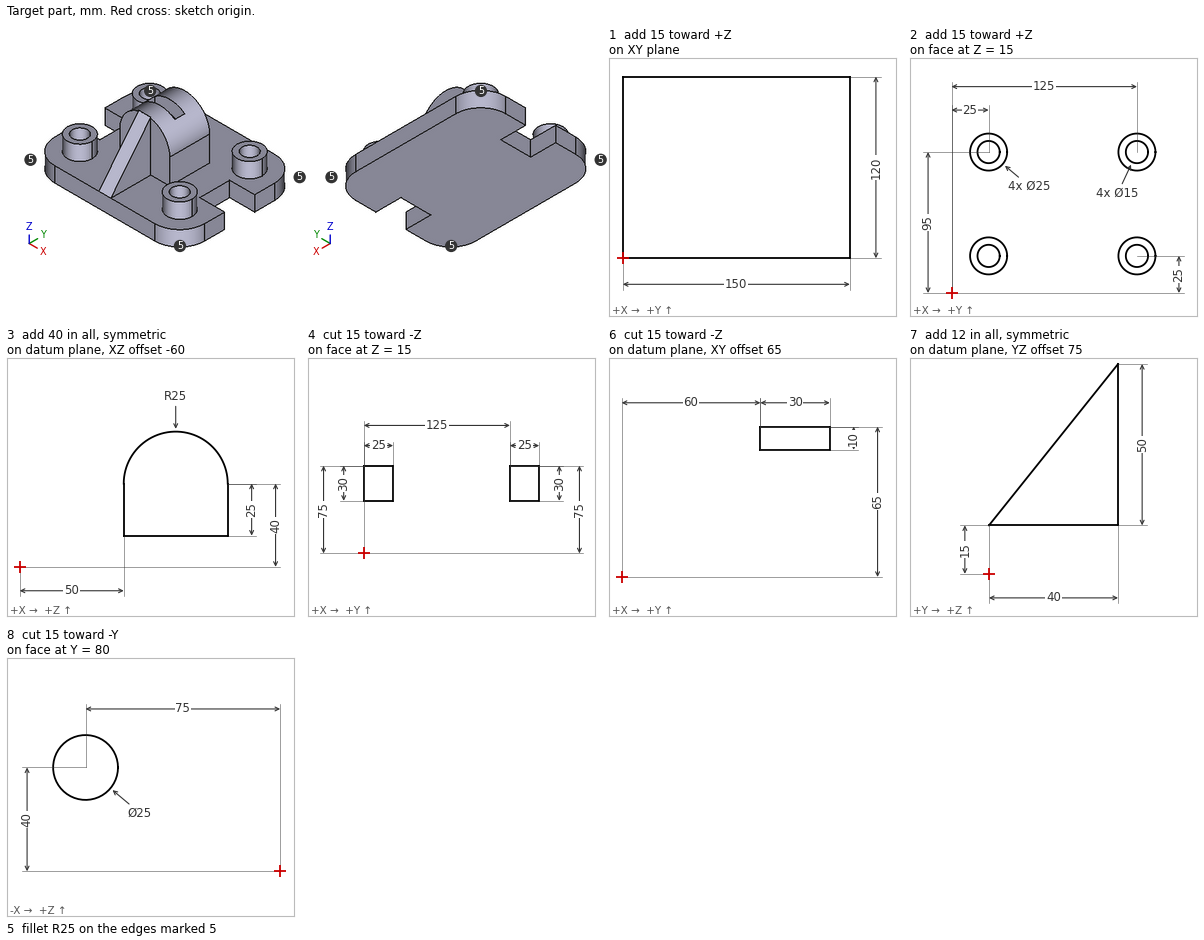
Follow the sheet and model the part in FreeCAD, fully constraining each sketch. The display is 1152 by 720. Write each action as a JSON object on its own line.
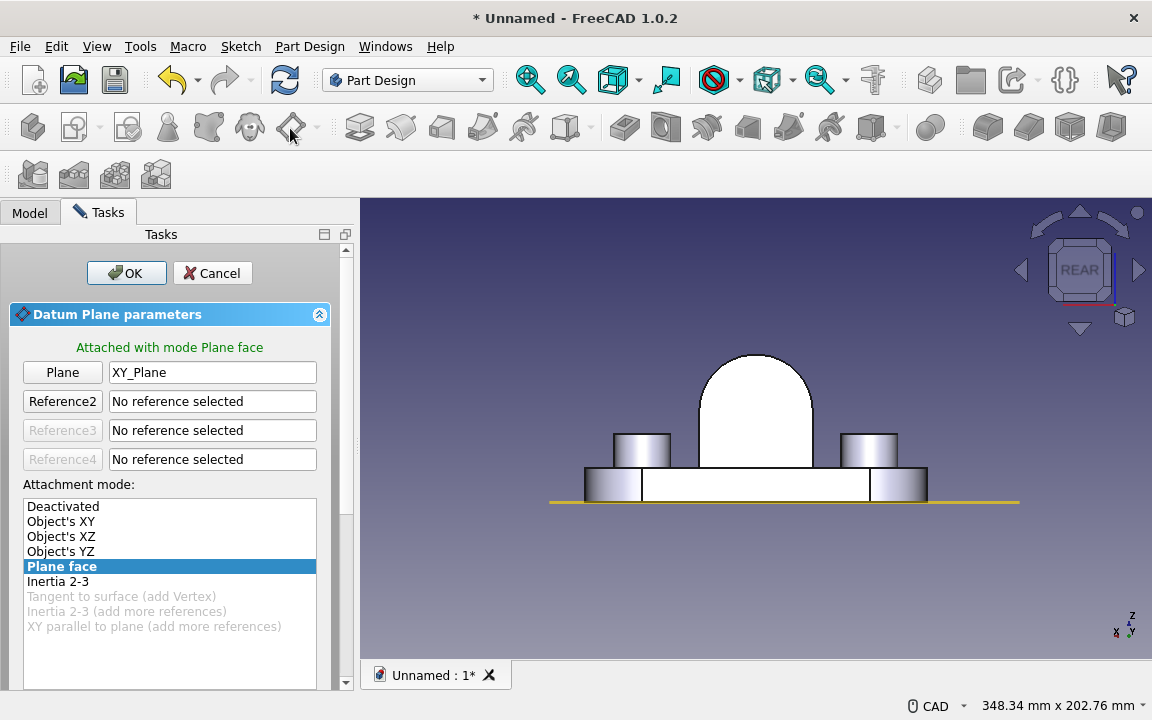
{"action": "scroll", "coordinate": [346, 467], "scroll_direction": "down", "scroll_amount": 4}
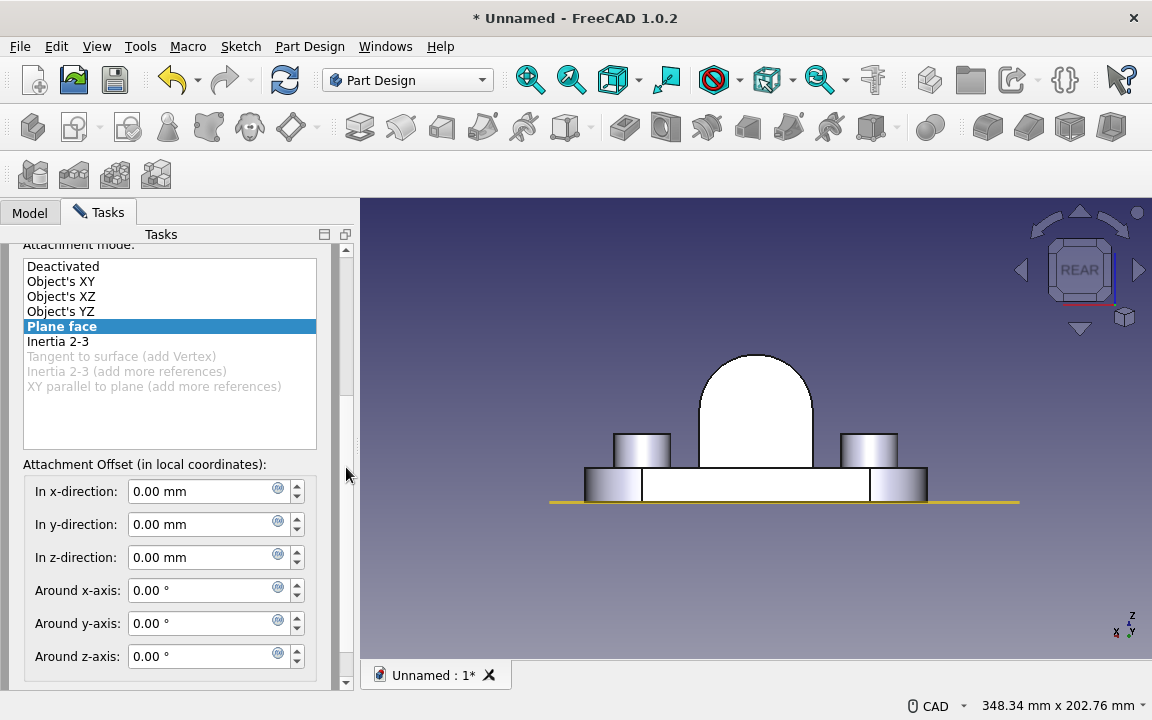
{"action": "triple_click", "coordinate": [210, 558]}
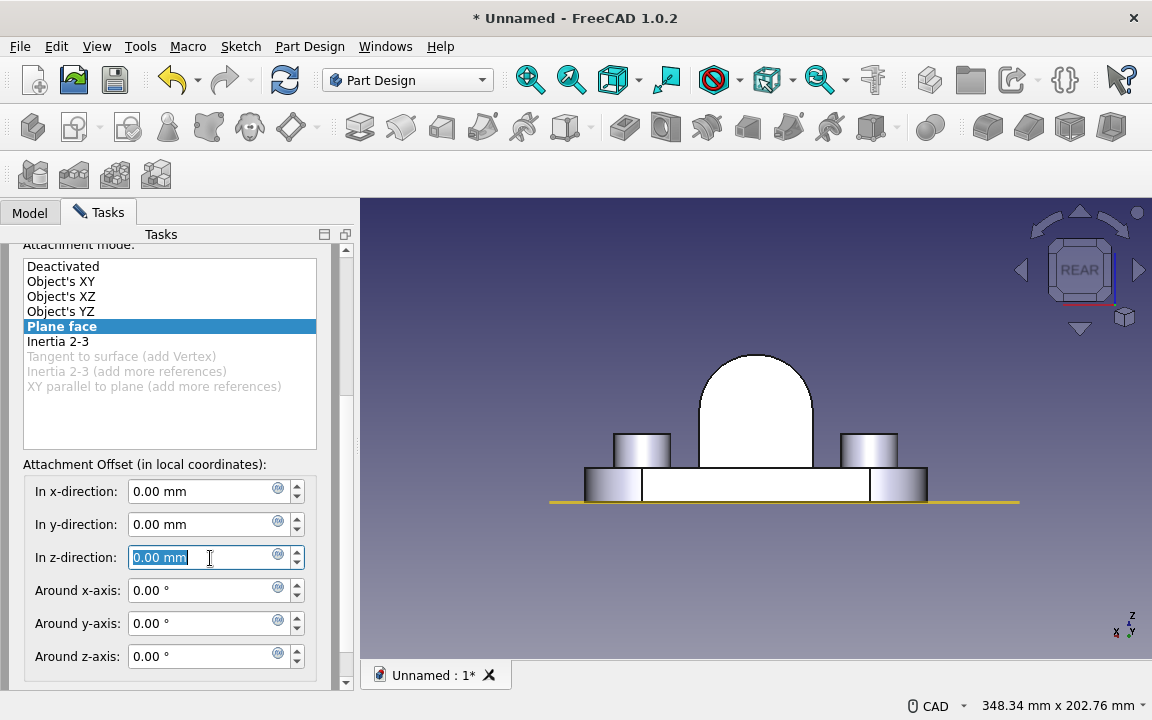
{"action": "type", "text": "65"}
{"action": "key", "text": "Tab"}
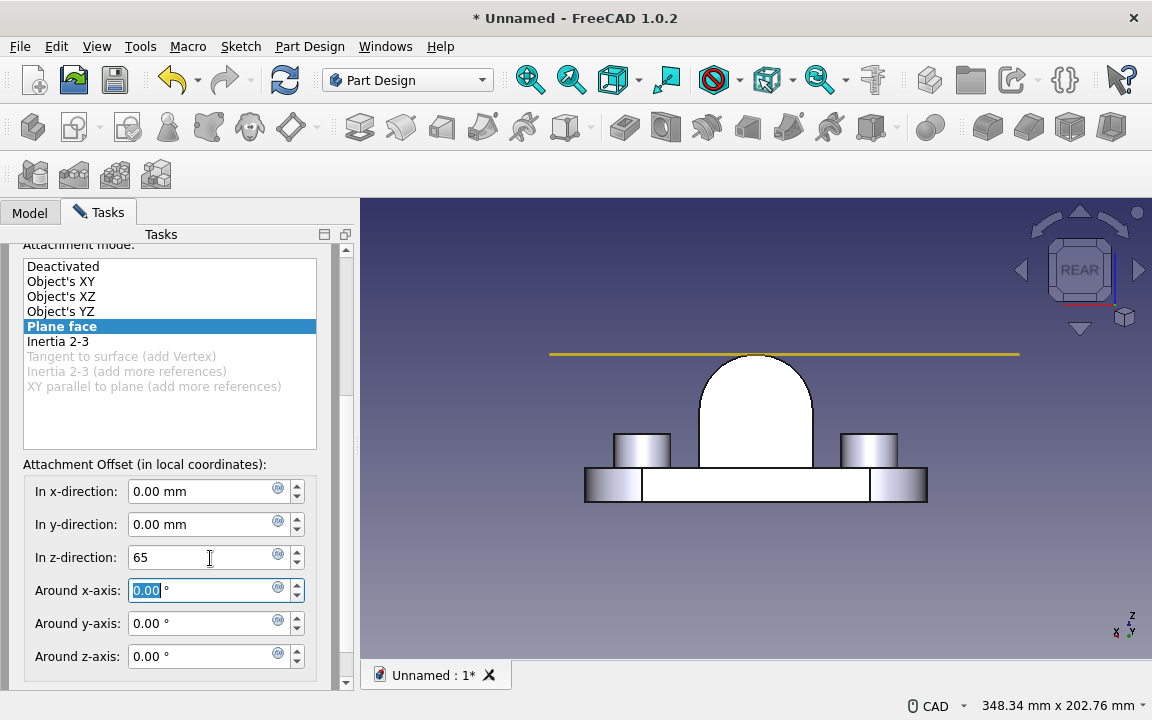
{"action": "scroll", "coordinate": [346, 467], "scroll_direction": "up", "scroll_amount": 5}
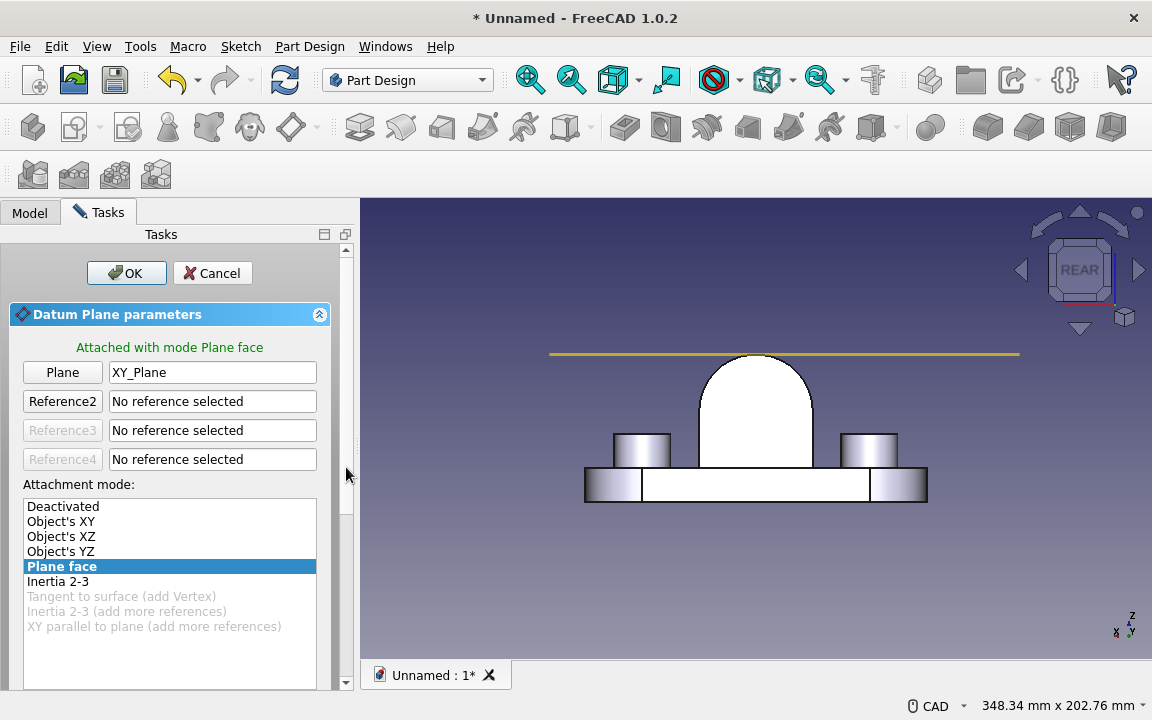
{"action": "left_click", "coordinate": [127, 273]}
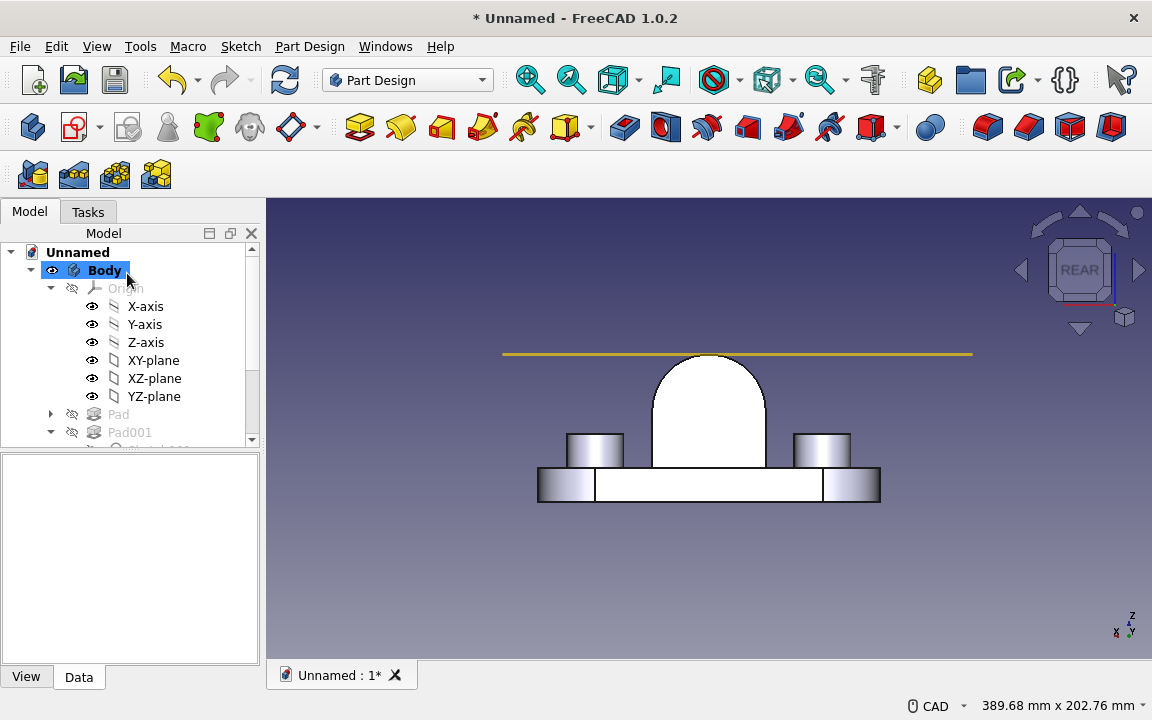
{"action": "scroll", "coordinate": [101, 338], "scroll_direction": "down", "scroll_amount": 3}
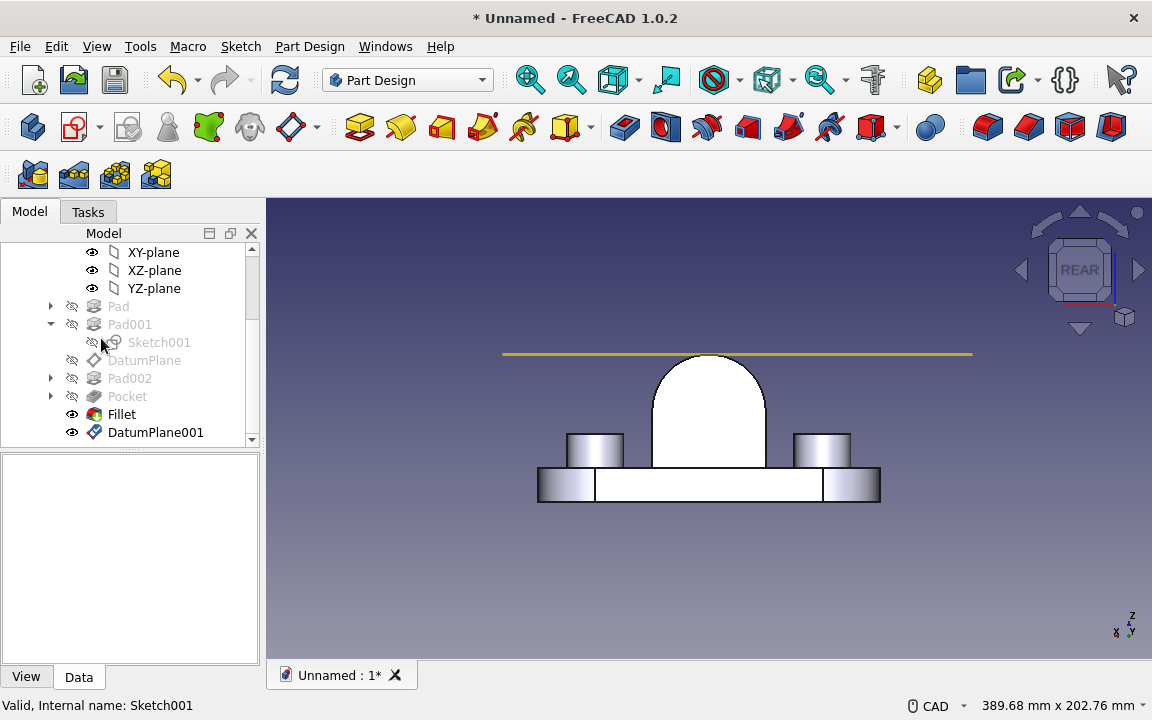
{"action": "left_click", "coordinate": [117, 432]}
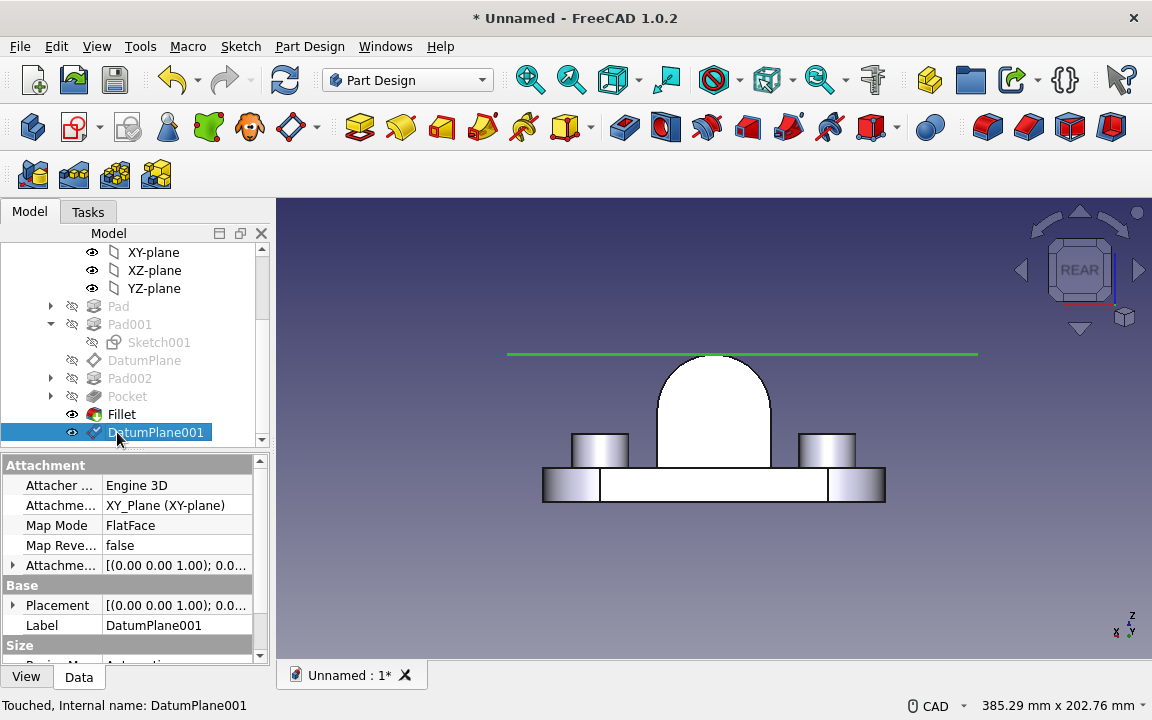
{"action": "left_click", "coordinate": [74, 128]}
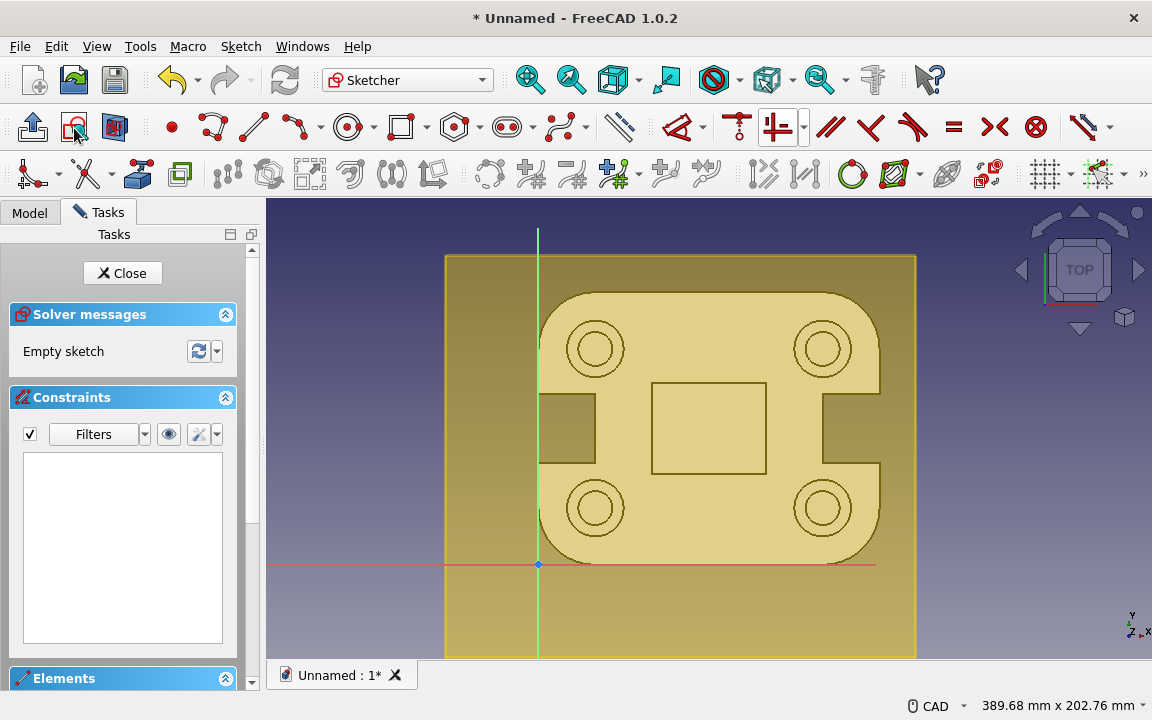
{"action": "scroll", "coordinate": [720, 429], "scroll_direction": "up", "scroll_amount": 10}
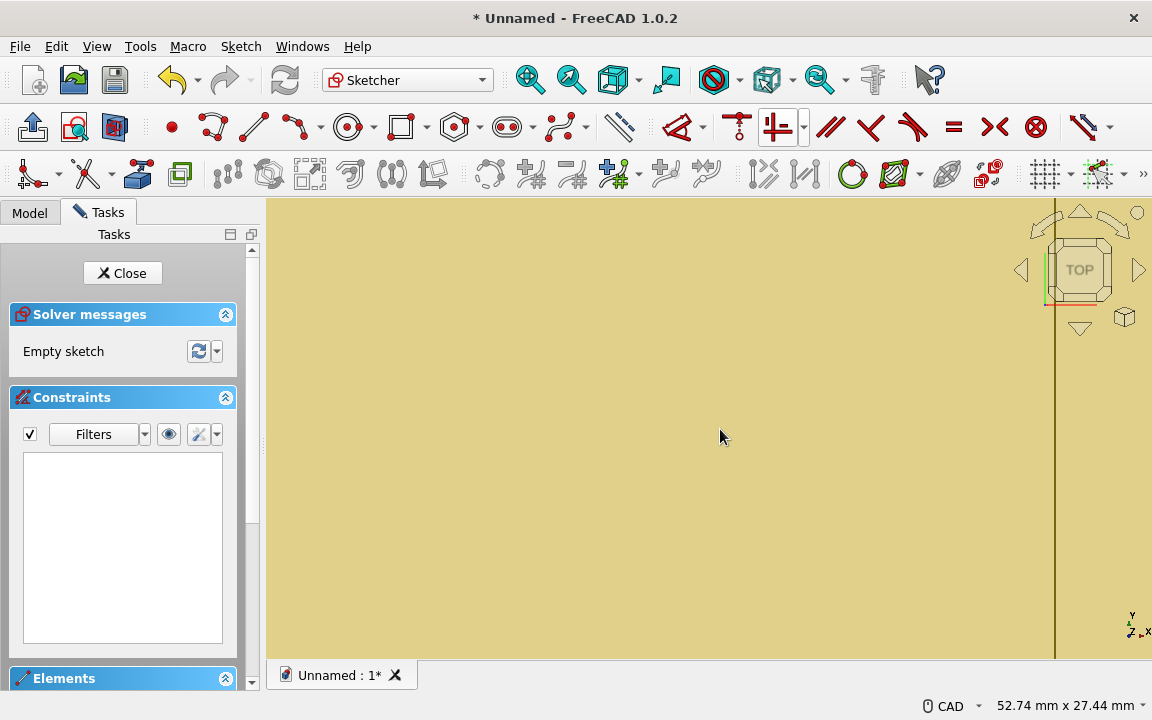
{"action": "left_click", "coordinate": [400, 128]}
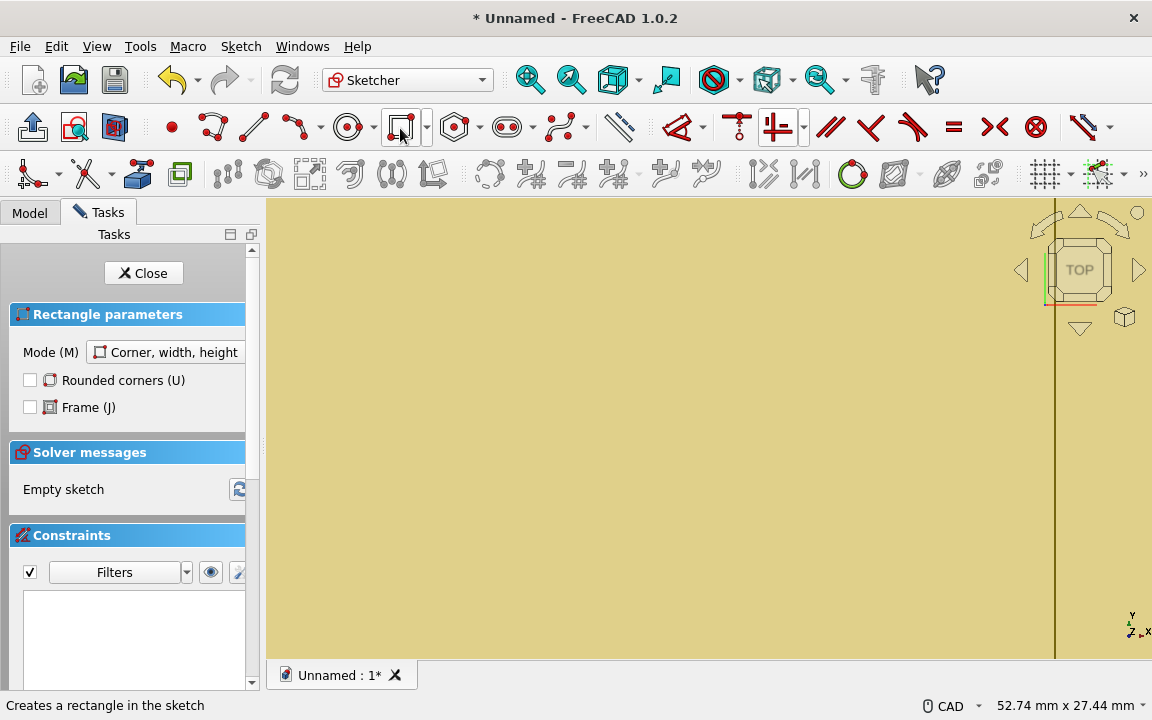
{"action": "left_click", "coordinate": [383, 338]}
{"action": "left_click", "coordinate": [887, 506]}
{"action": "key", "text": "Escape"}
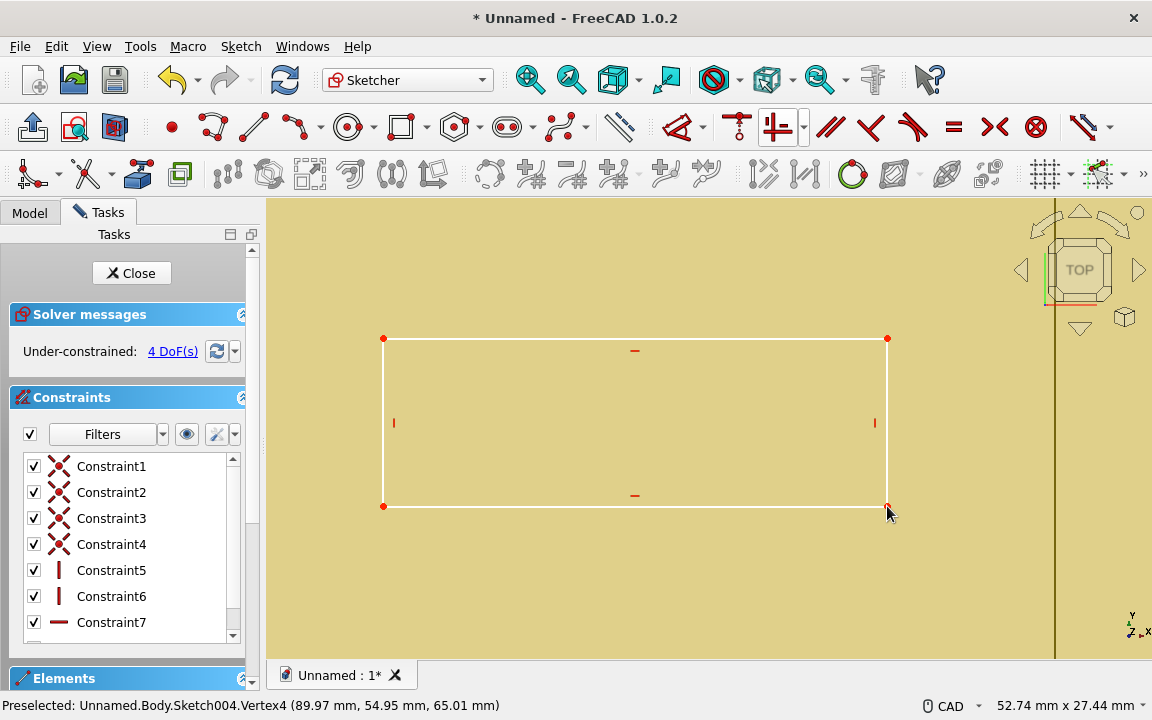
{"action": "left_click", "coordinate": [676, 128]}